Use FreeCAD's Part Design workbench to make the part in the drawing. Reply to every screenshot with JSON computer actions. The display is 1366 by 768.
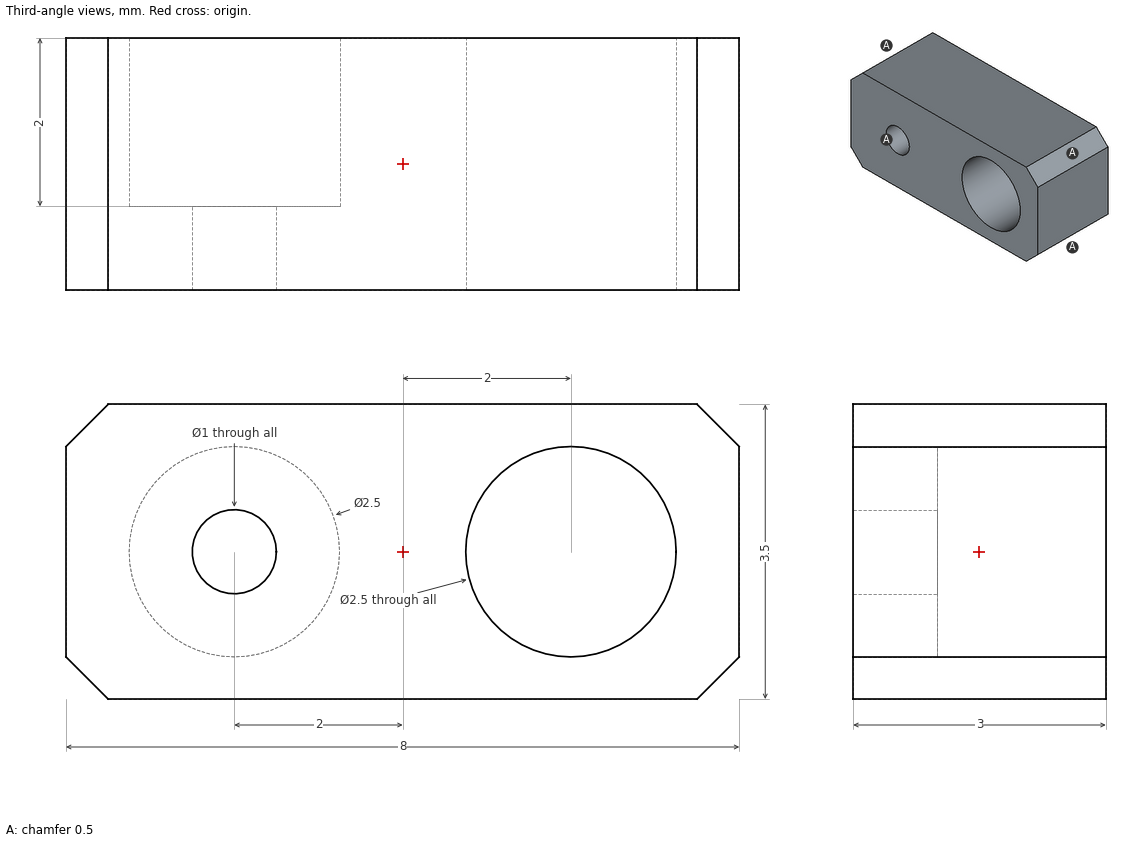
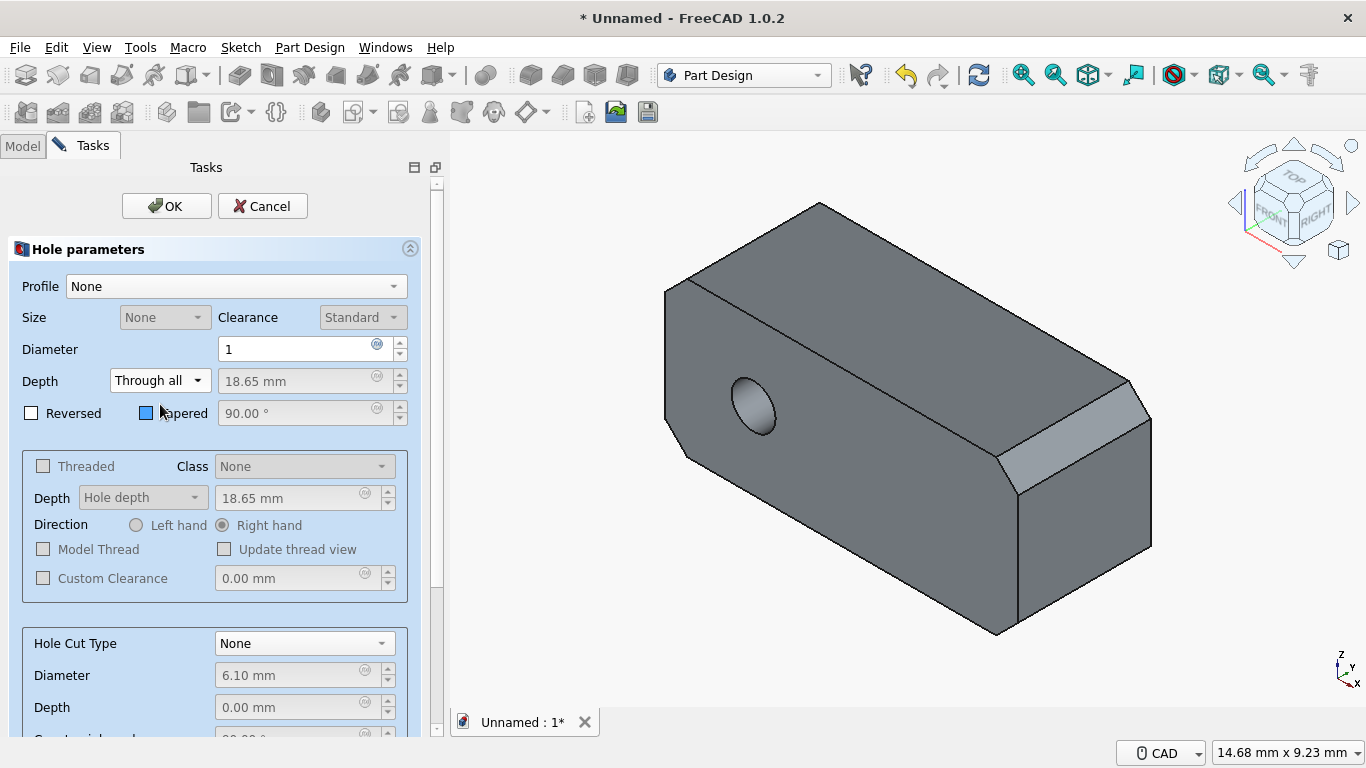
{"action": "left_click", "coordinate": [167, 206]}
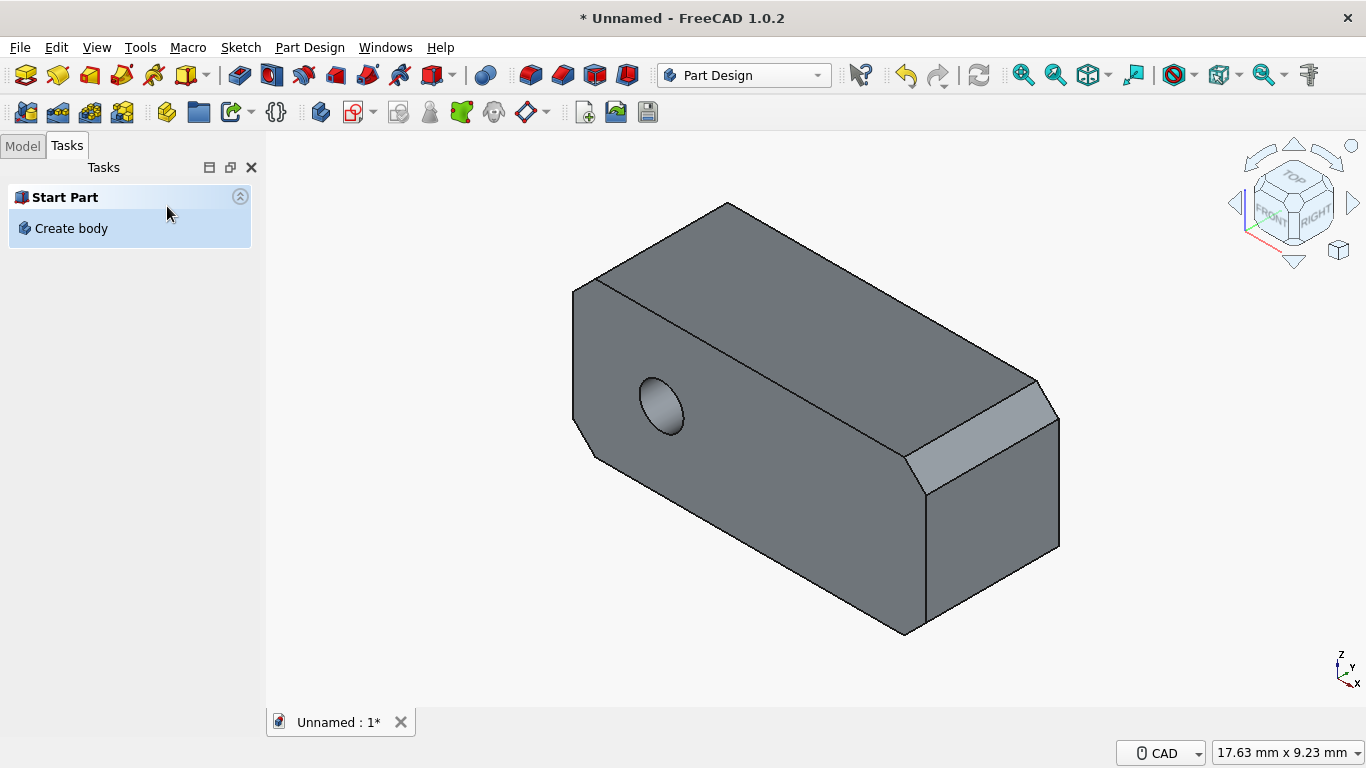
{"action": "left_click", "coordinate": [800, 485]}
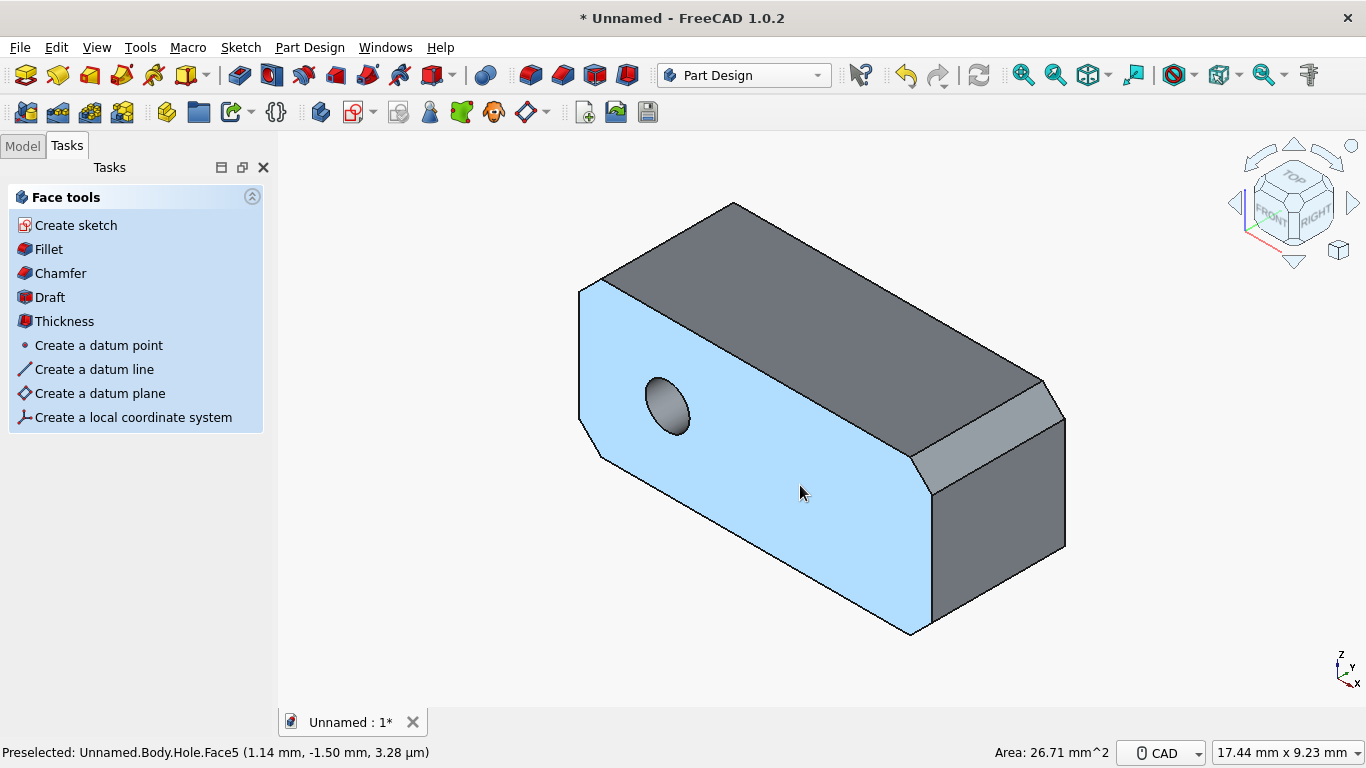
{"action": "left_click", "coordinate": [354, 112]}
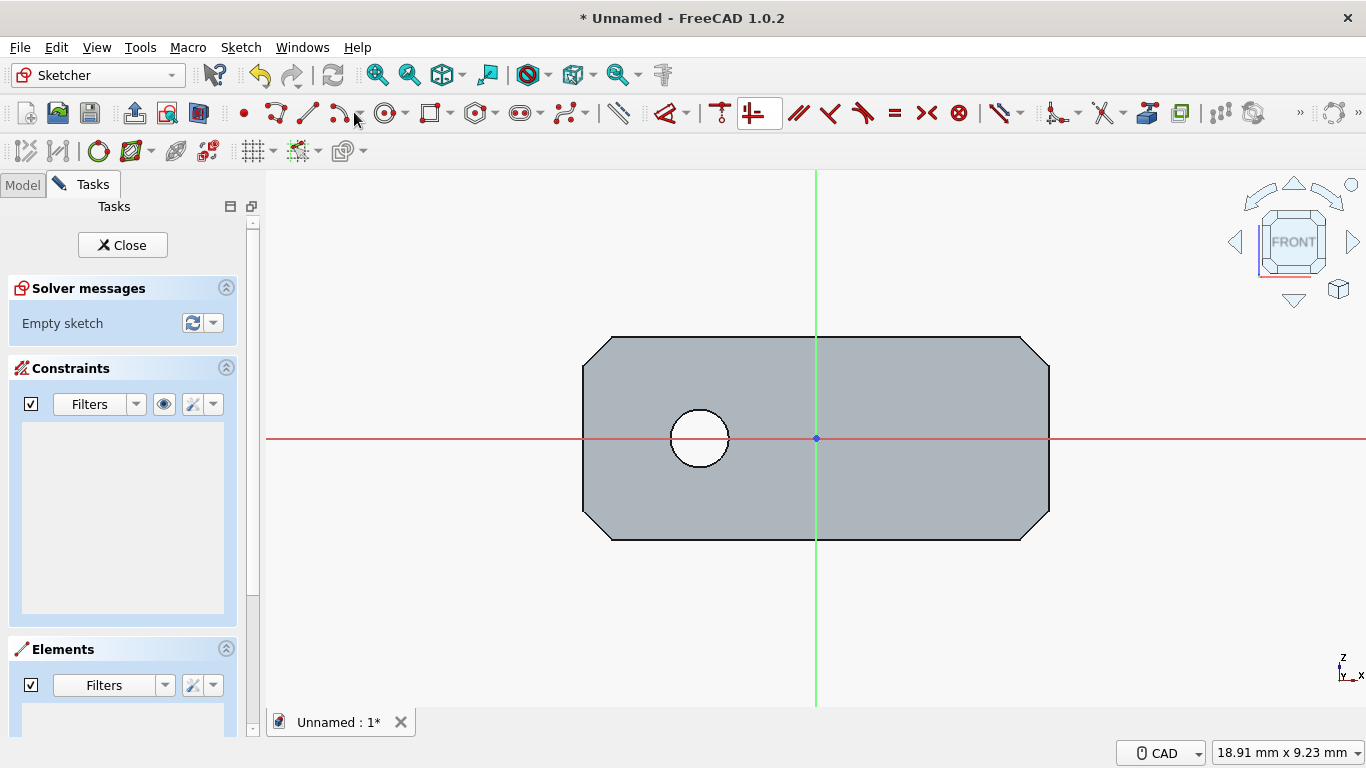
{"action": "scroll", "coordinate": [1044, 438], "scroll_direction": "up", "scroll_amount": 4}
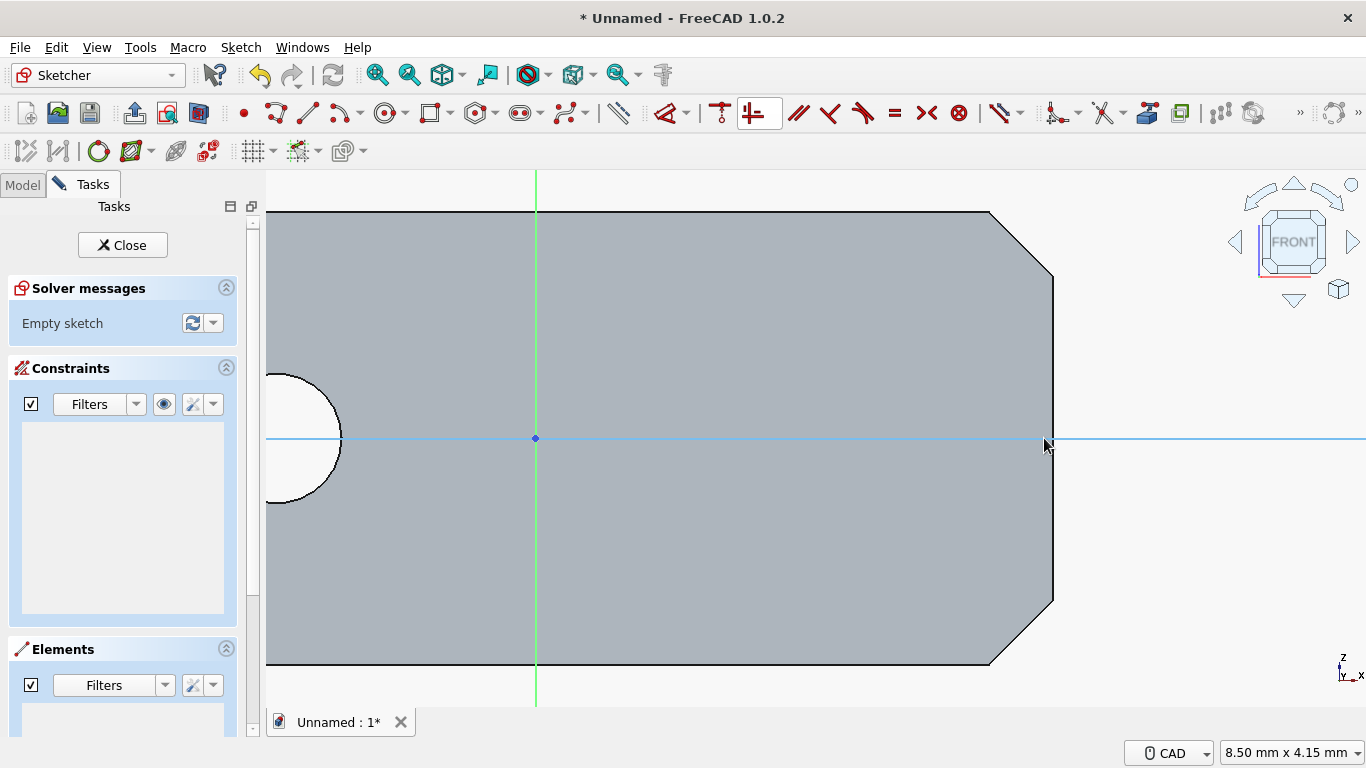
{"action": "left_click", "coordinate": [386, 114]}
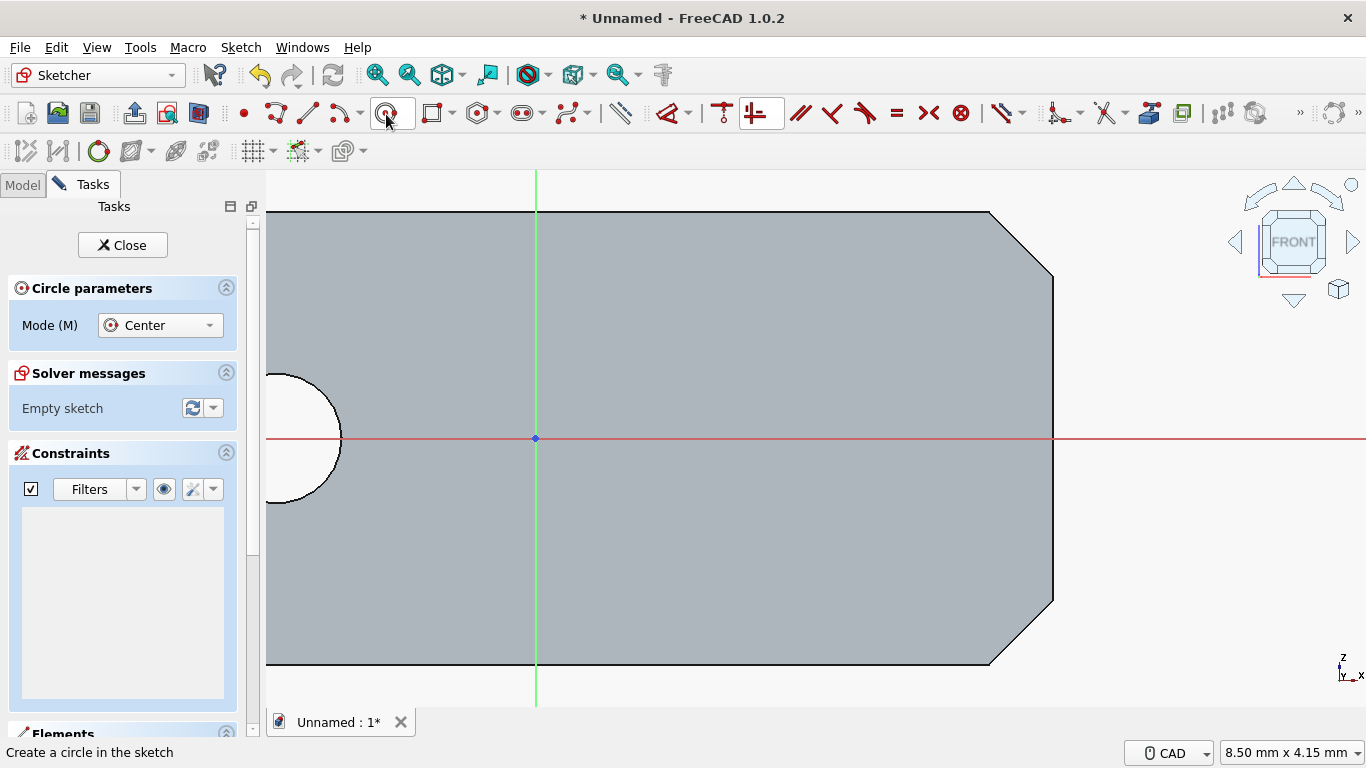
{"action": "left_click", "coordinate": [795, 438]}
{"action": "left_click", "coordinate": [909, 324]}
{"action": "key", "text": "Escape"}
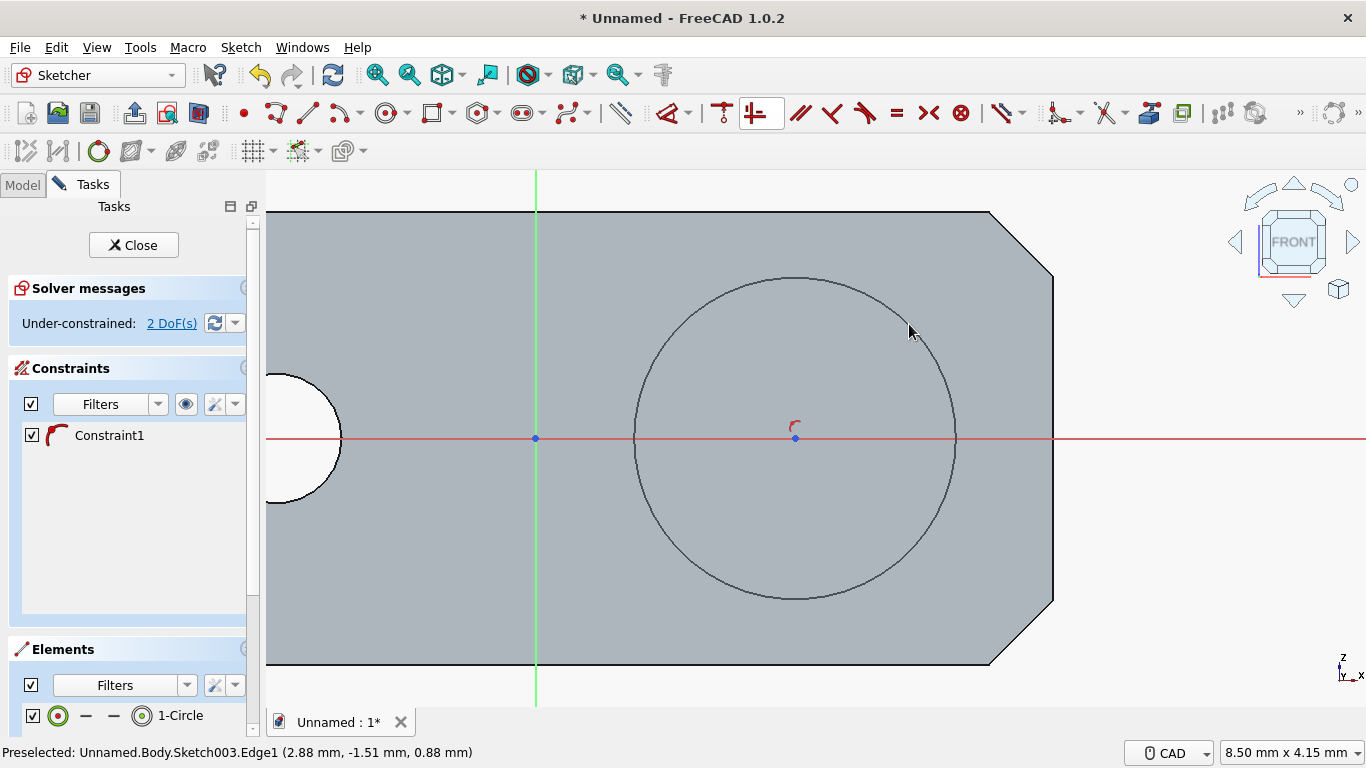
{"action": "left_click", "coordinate": [668, 114]}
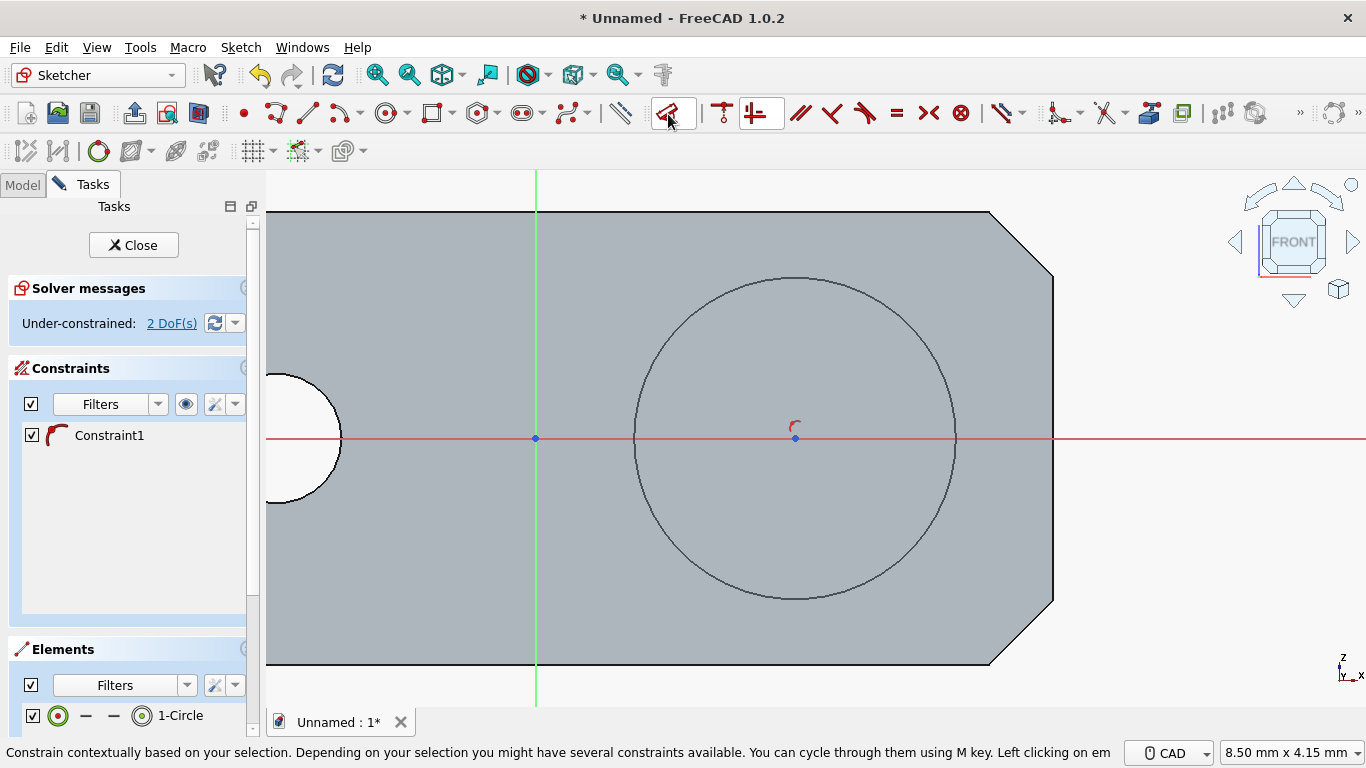
{"action": "left_click", "coordinate": [908, 324]}
{"action": "left_click", "coordinate": [930, 301]}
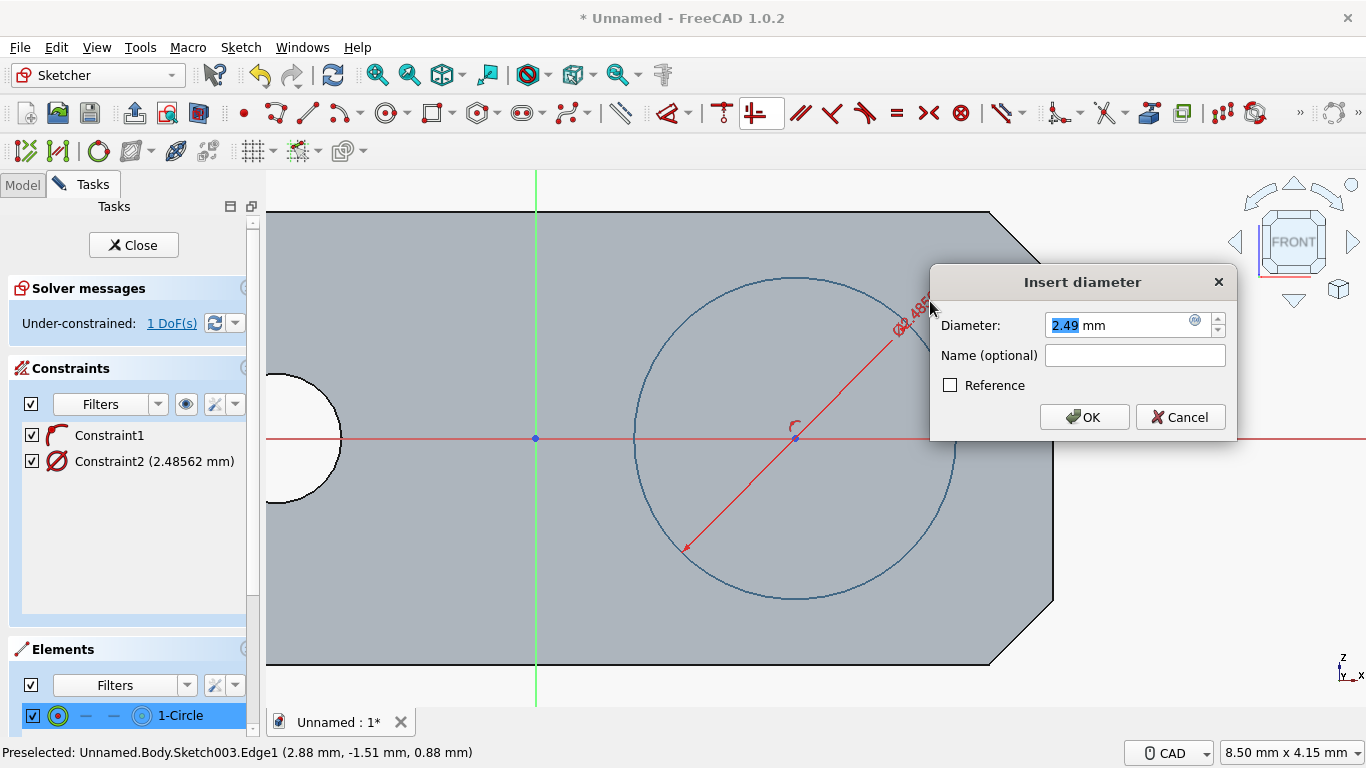
{"action": "type", "text": "2.5"}
{"action": "key", "text": "Return"}